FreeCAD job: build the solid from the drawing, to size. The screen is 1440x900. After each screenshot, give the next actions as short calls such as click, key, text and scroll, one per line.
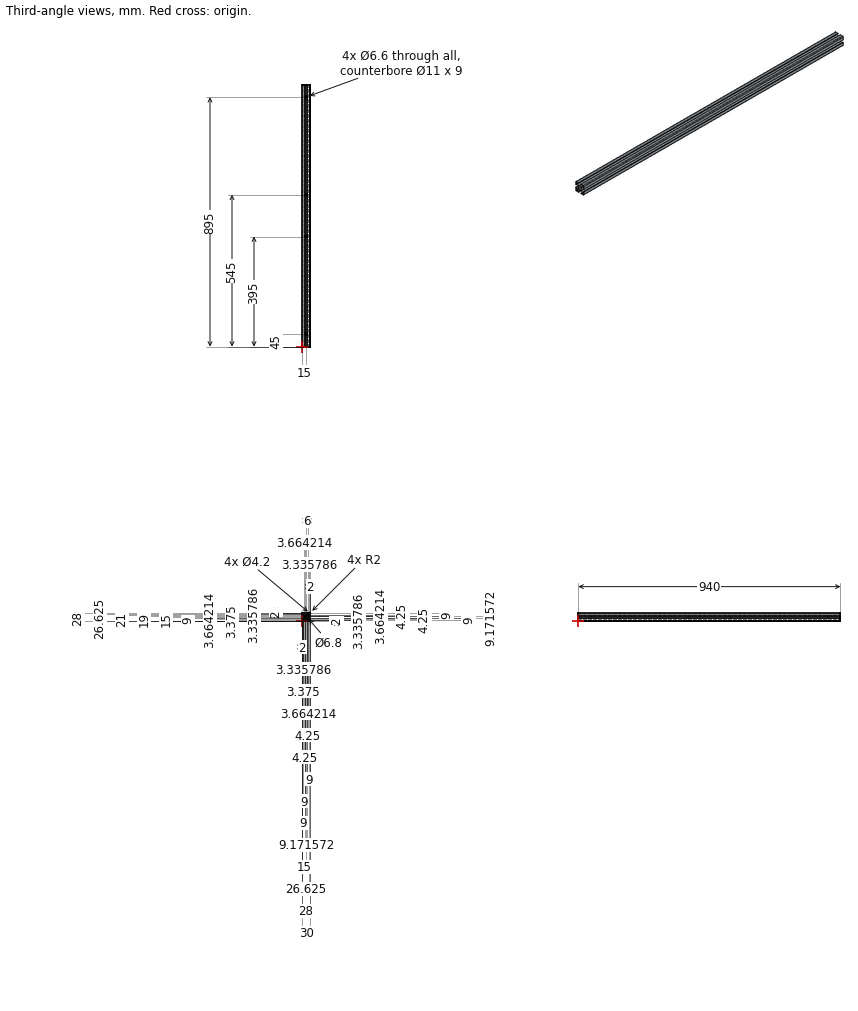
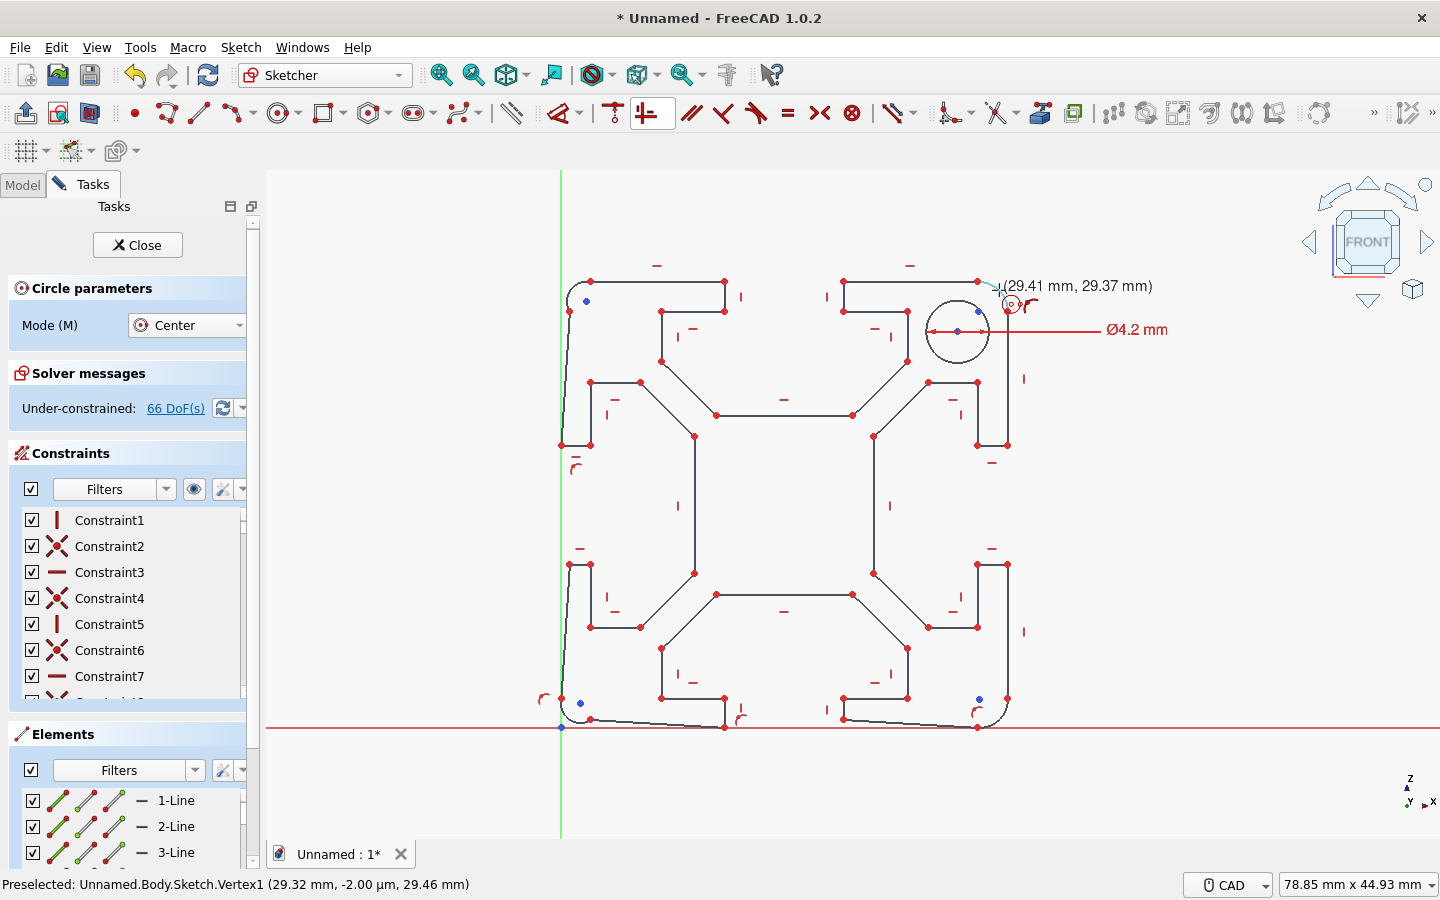
click(612, 331)
move(634, 309)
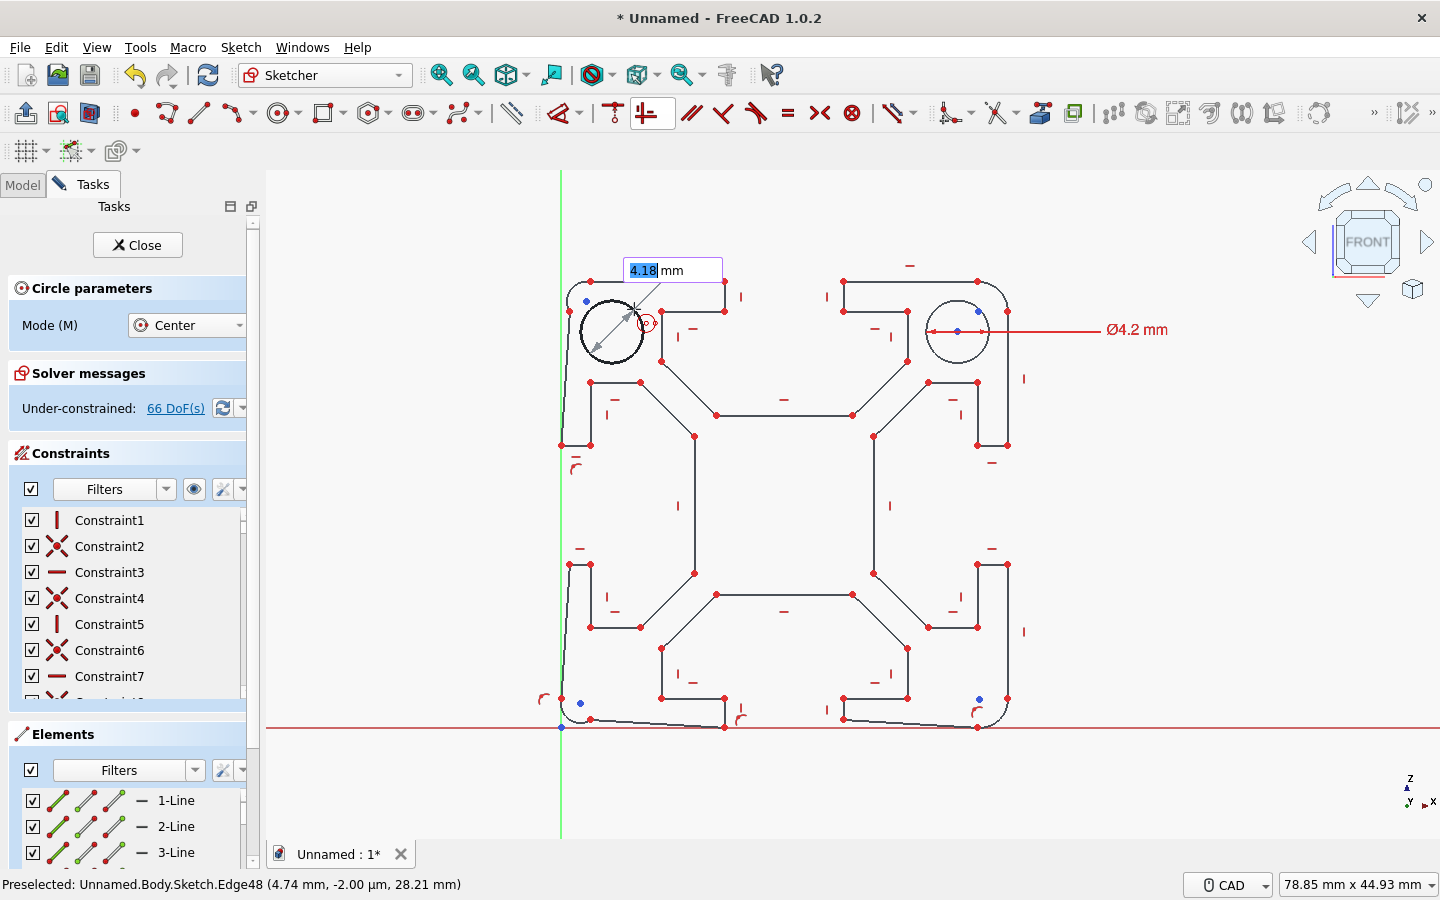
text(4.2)
key(Return)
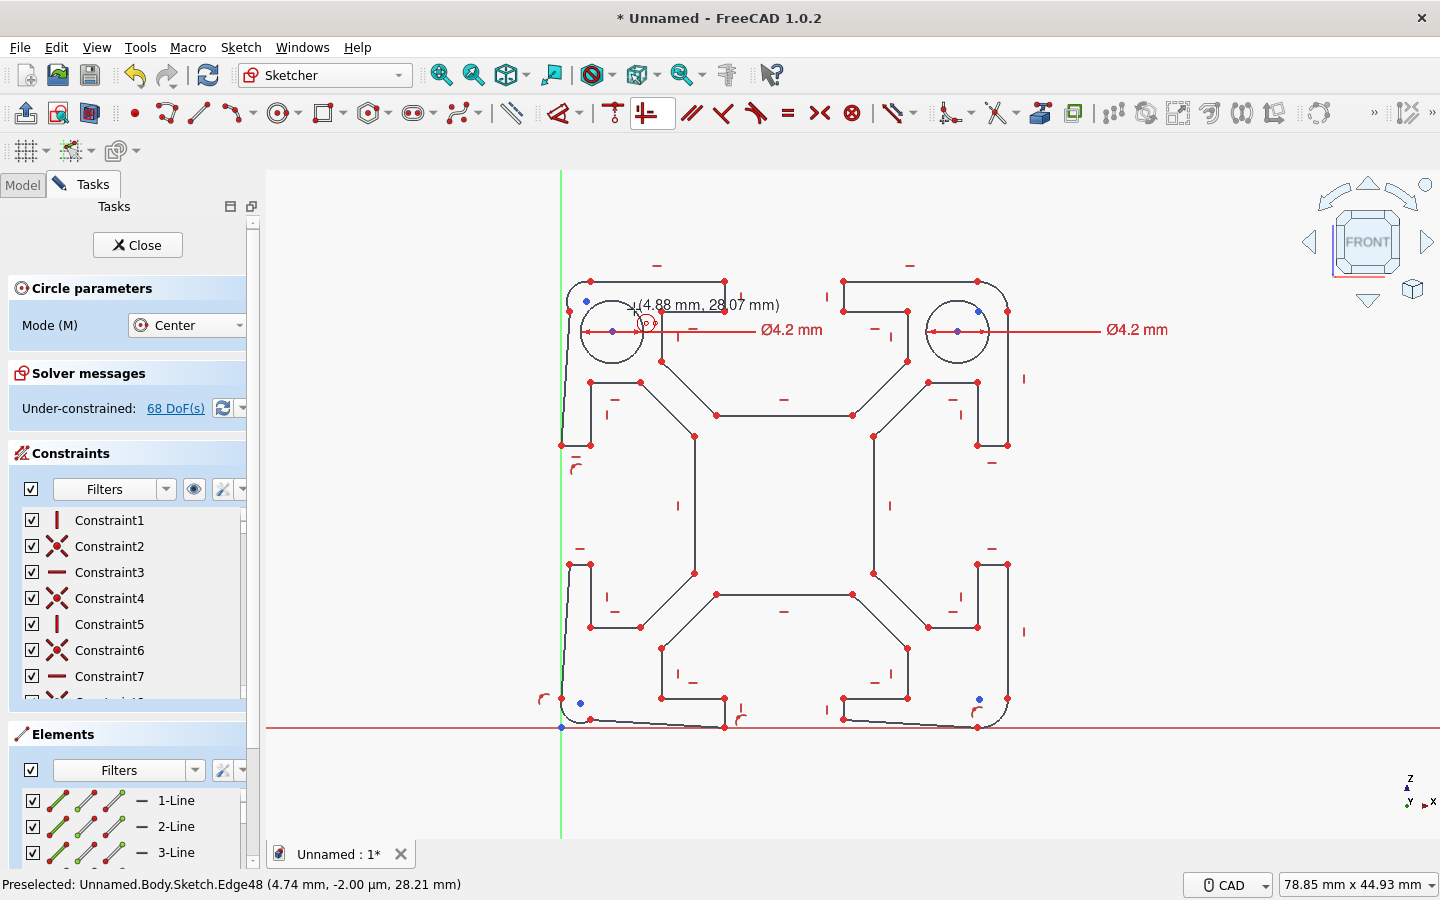
click(958, 678)
move(980, 656)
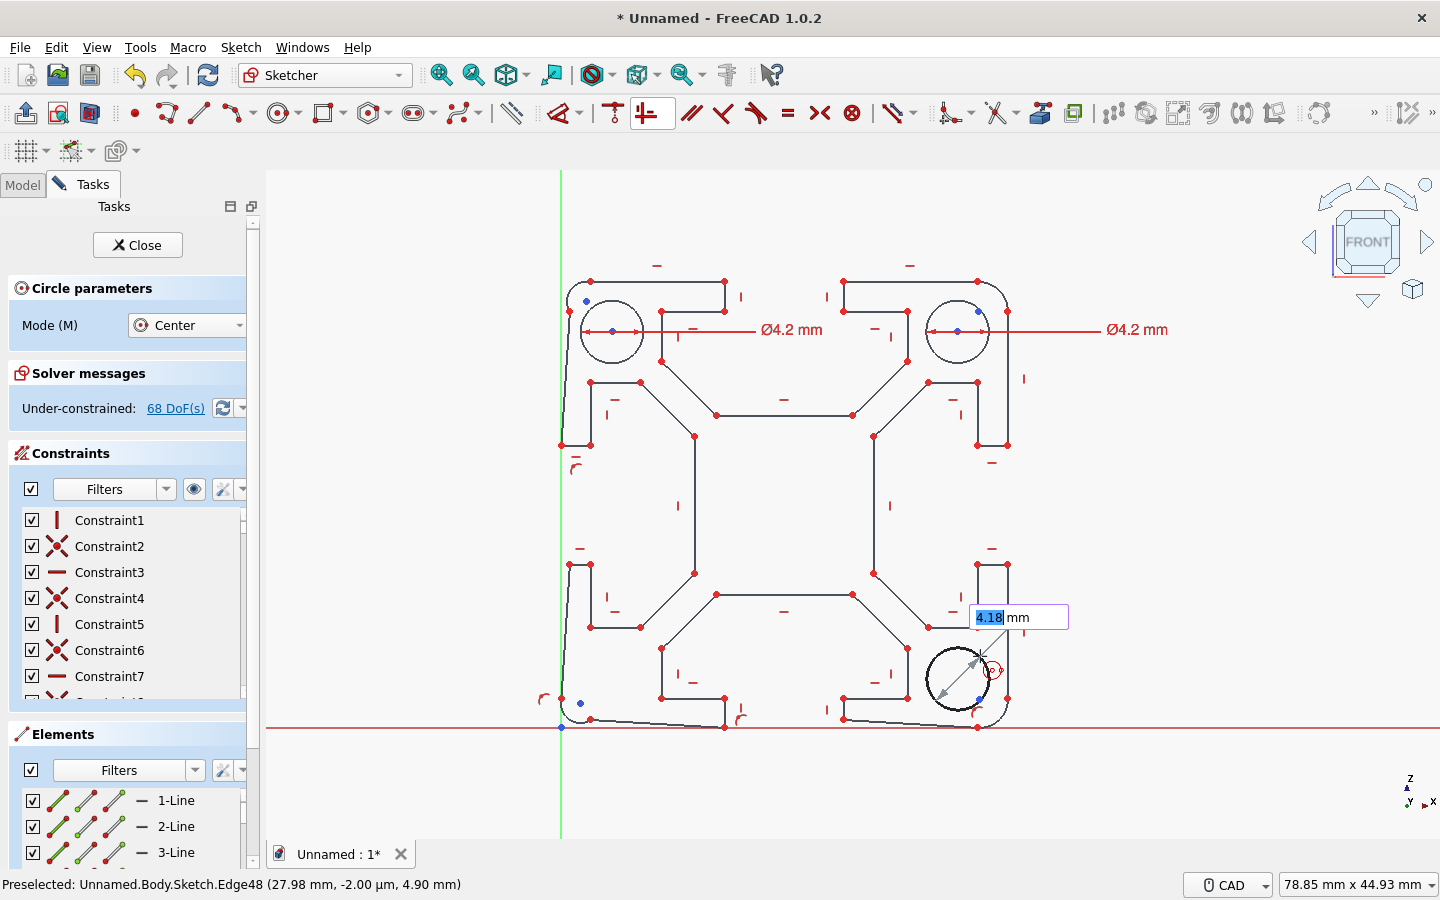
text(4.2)
key(Return)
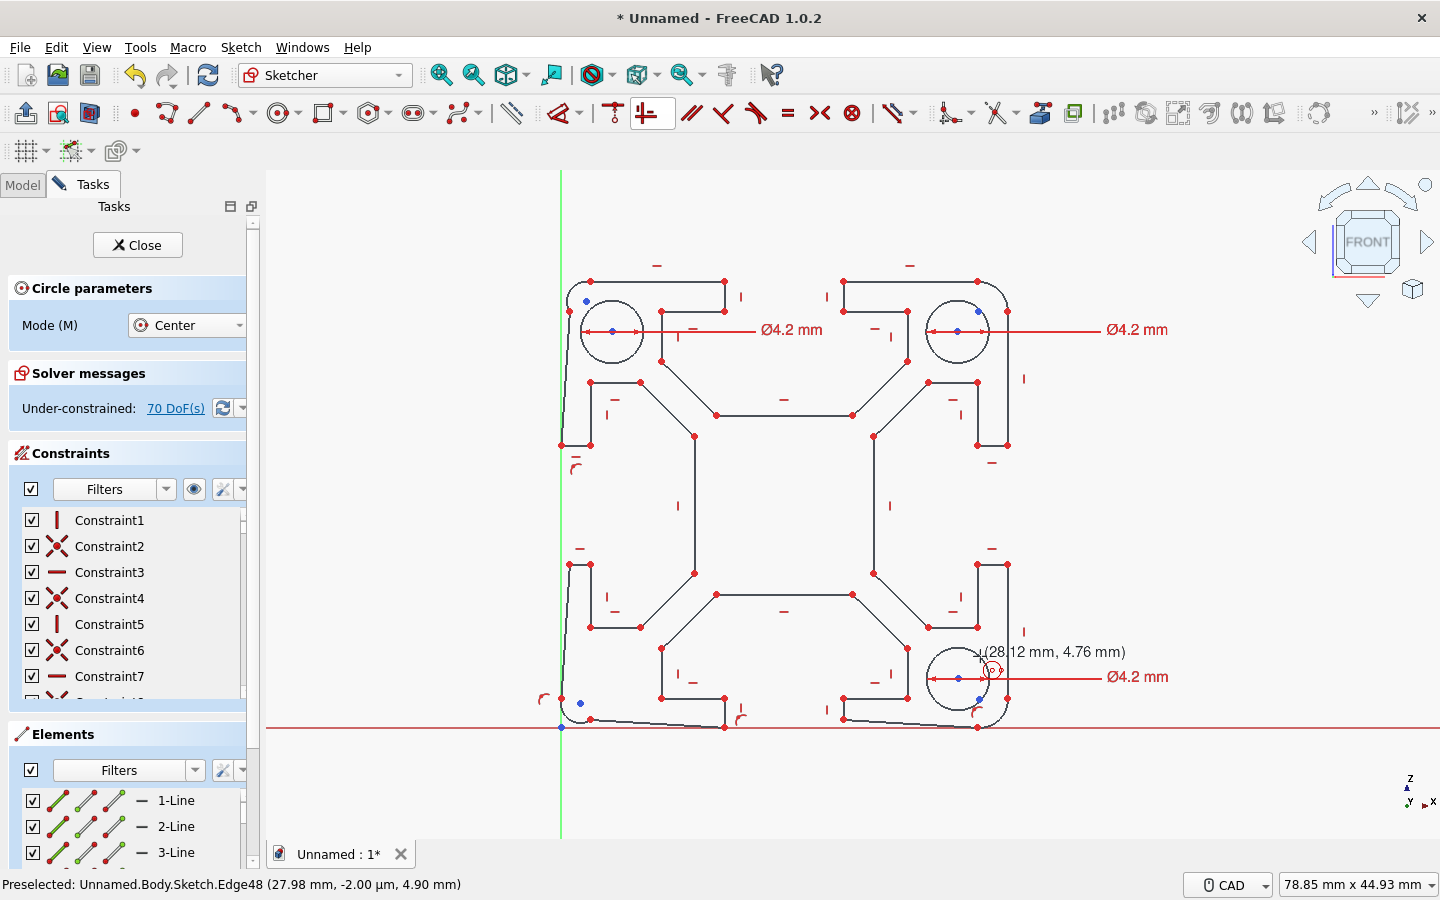
click(785, 505)
move(820, 469)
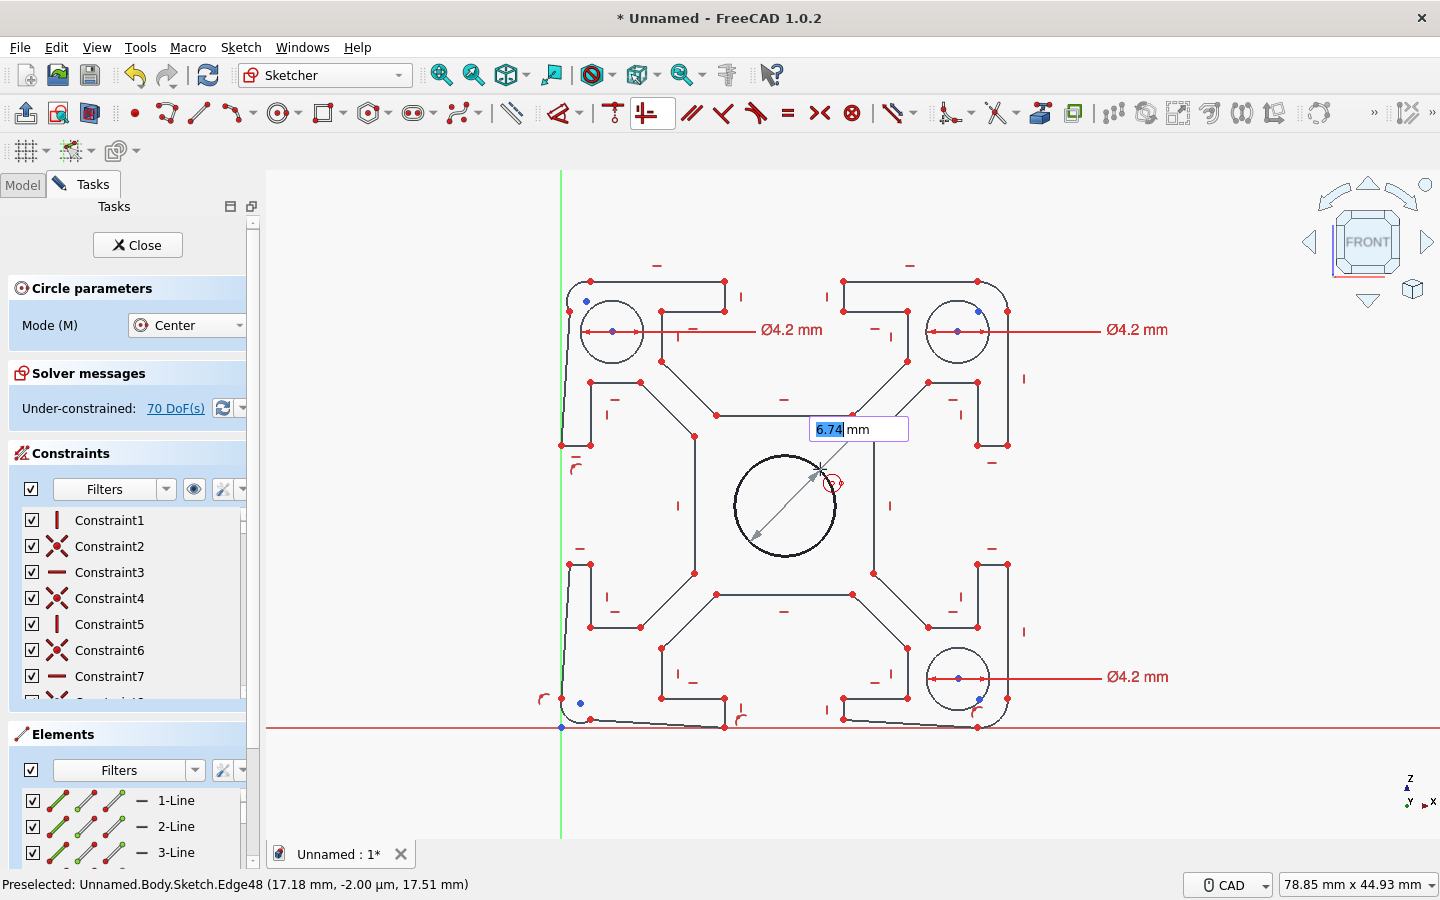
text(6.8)
key(Return)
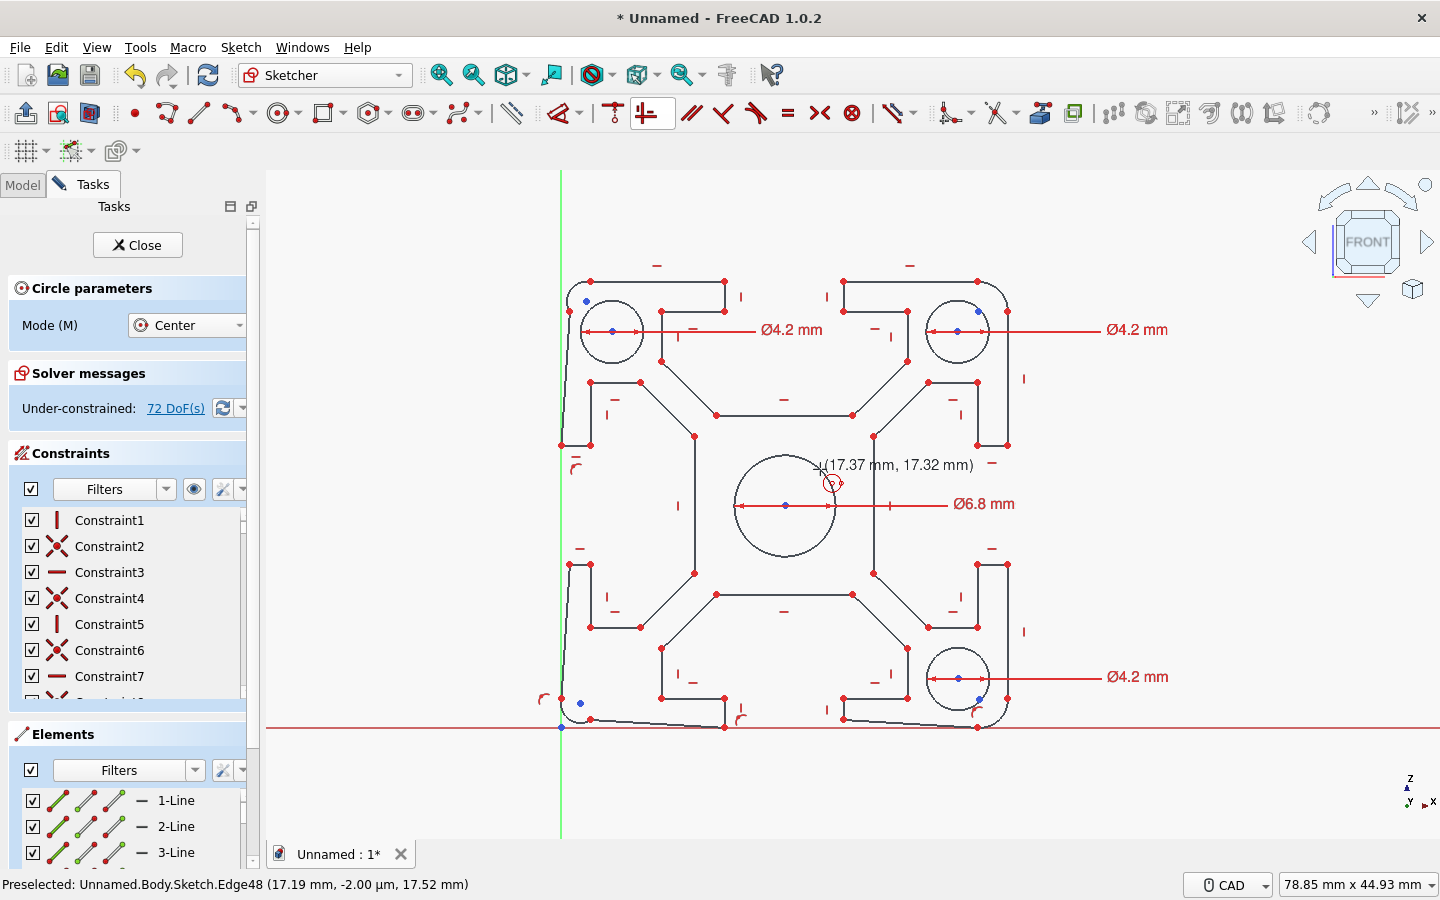
click(612, 678)
move(634, 656)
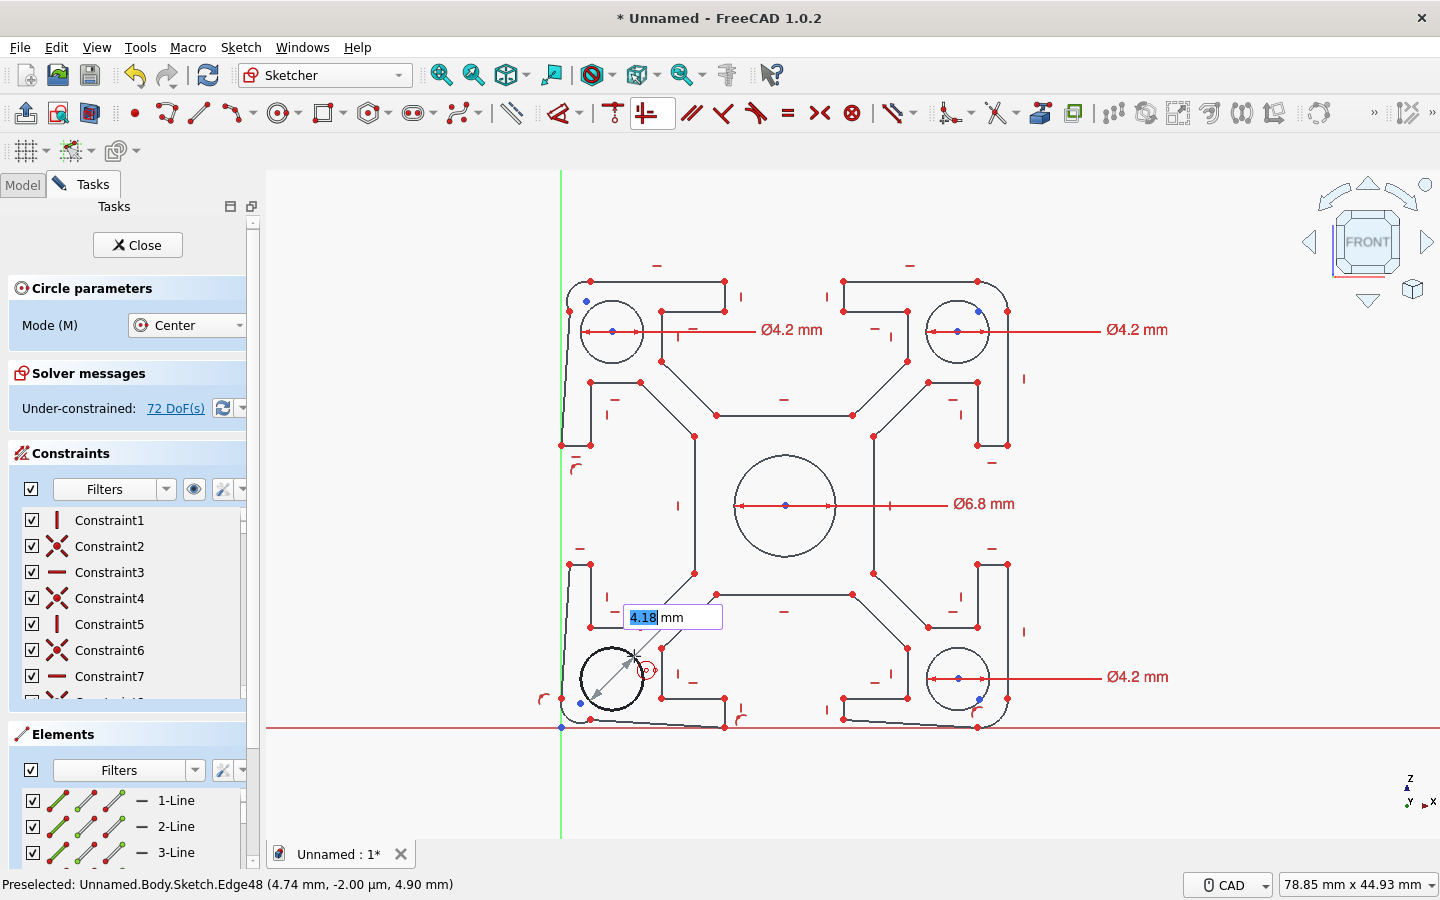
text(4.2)
key(Return)
key(Escape)